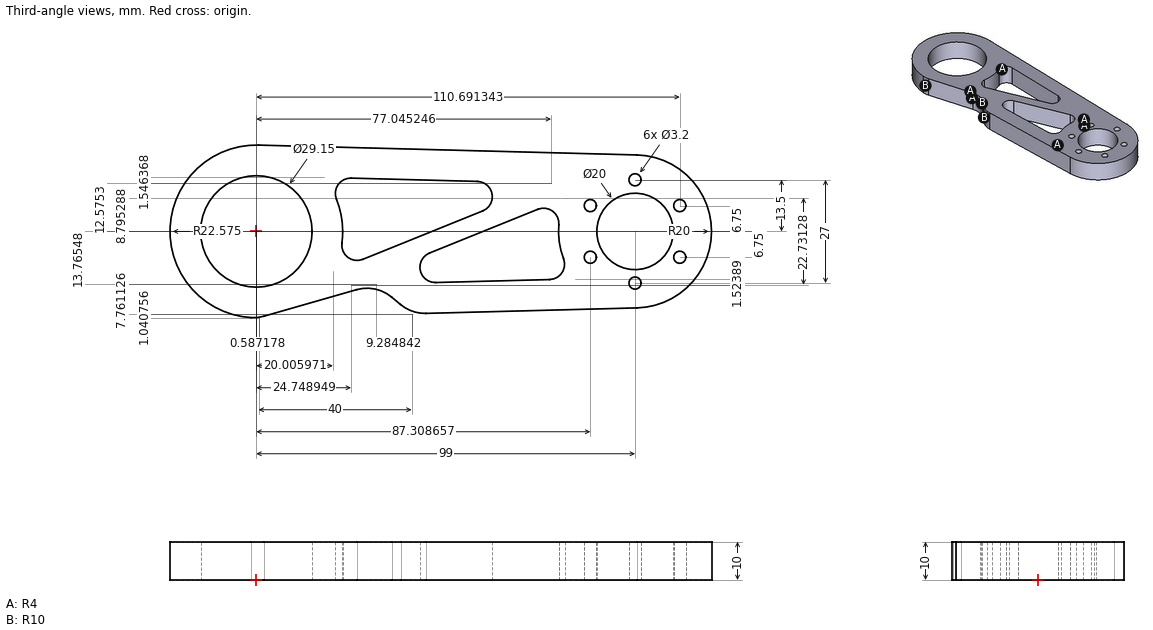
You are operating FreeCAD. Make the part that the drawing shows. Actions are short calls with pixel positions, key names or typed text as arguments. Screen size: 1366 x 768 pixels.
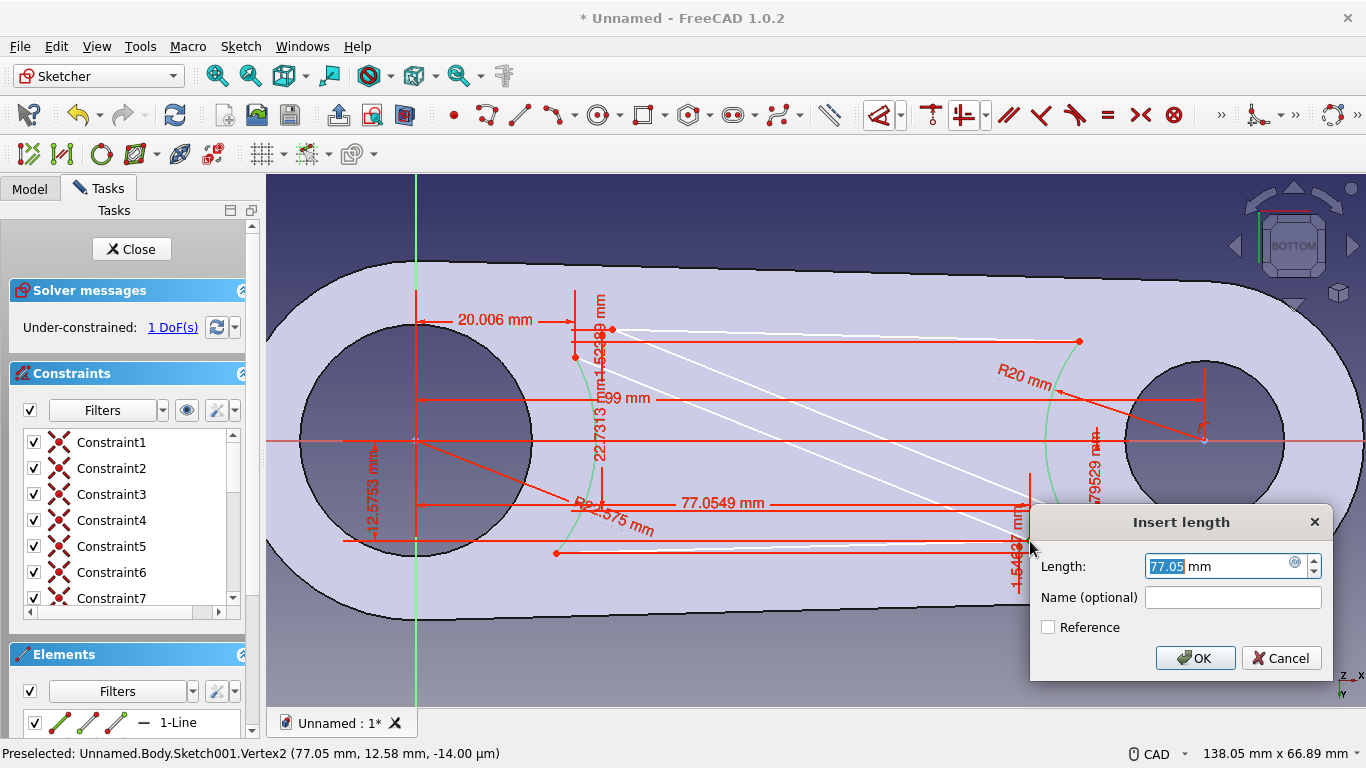
text(77.045246)
key(Return)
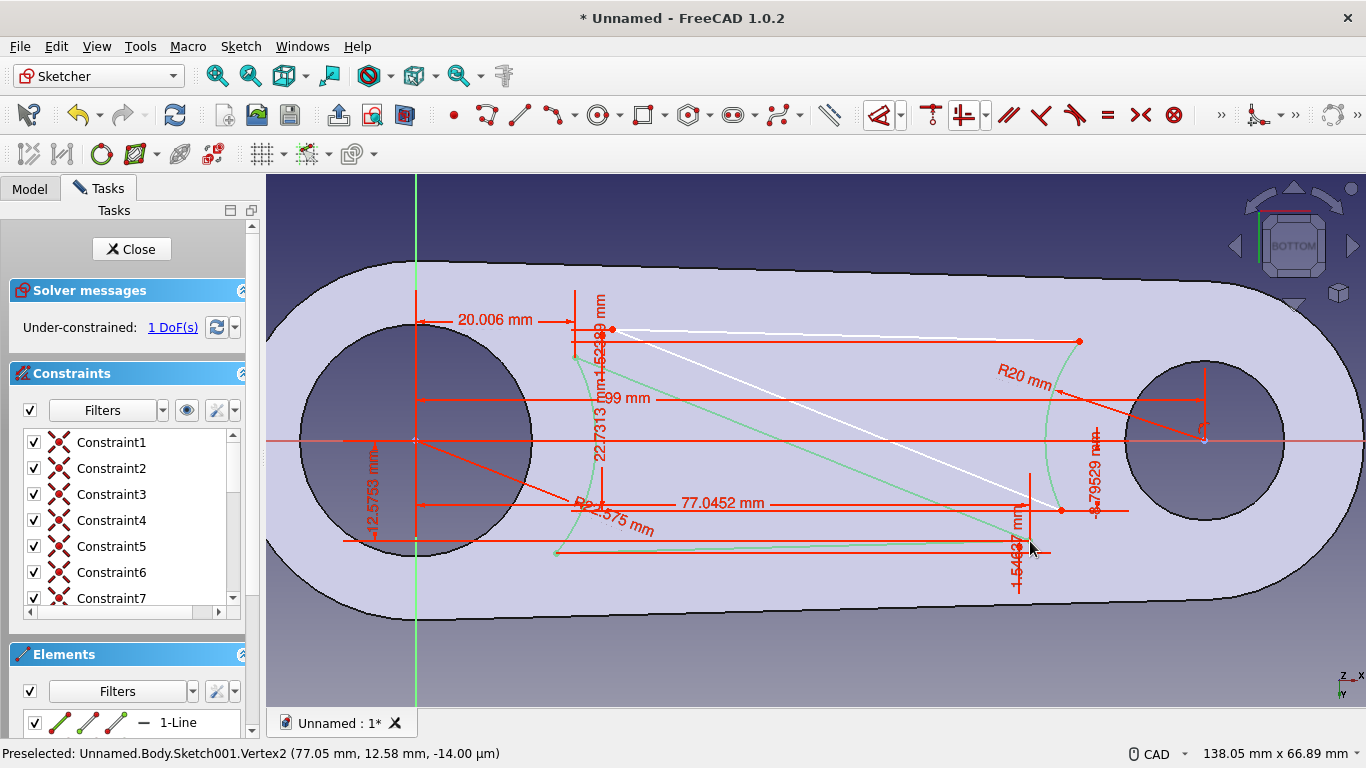
click(613, 330)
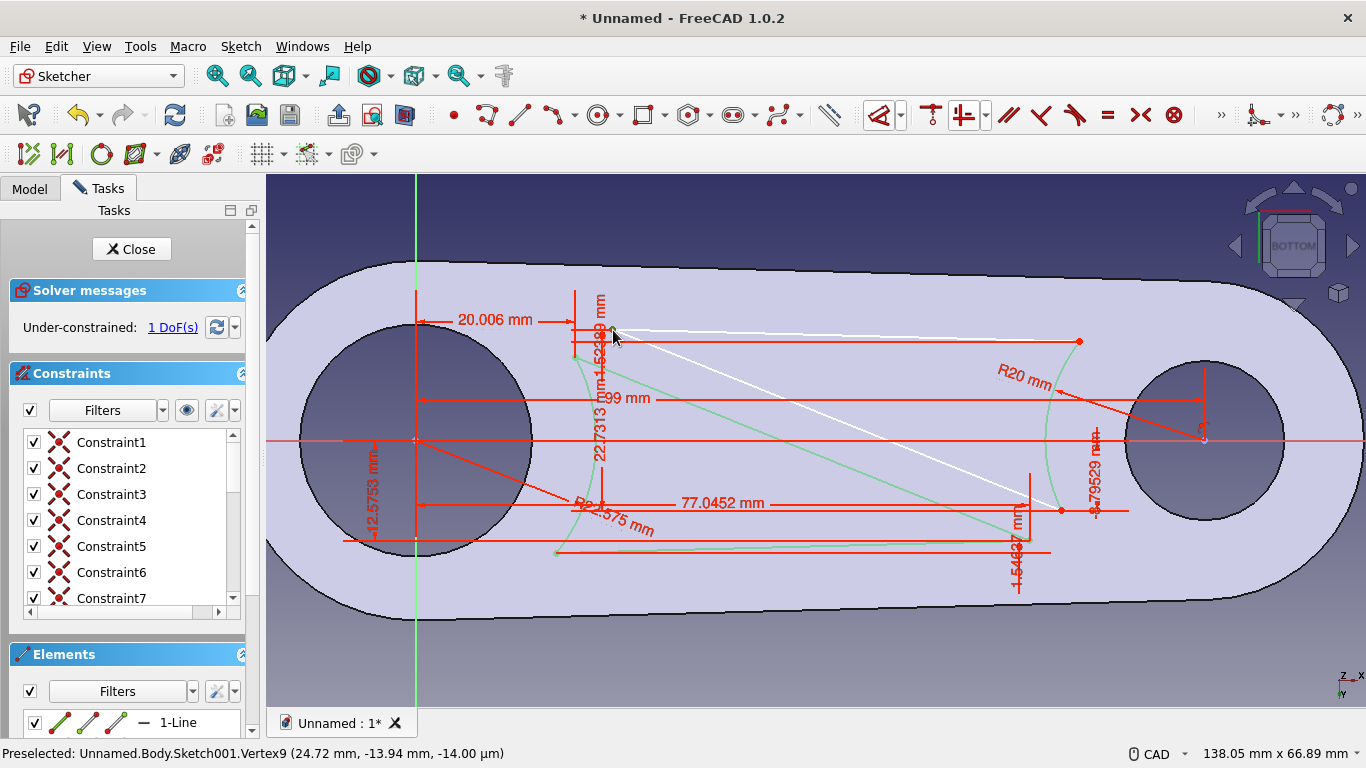
key(l)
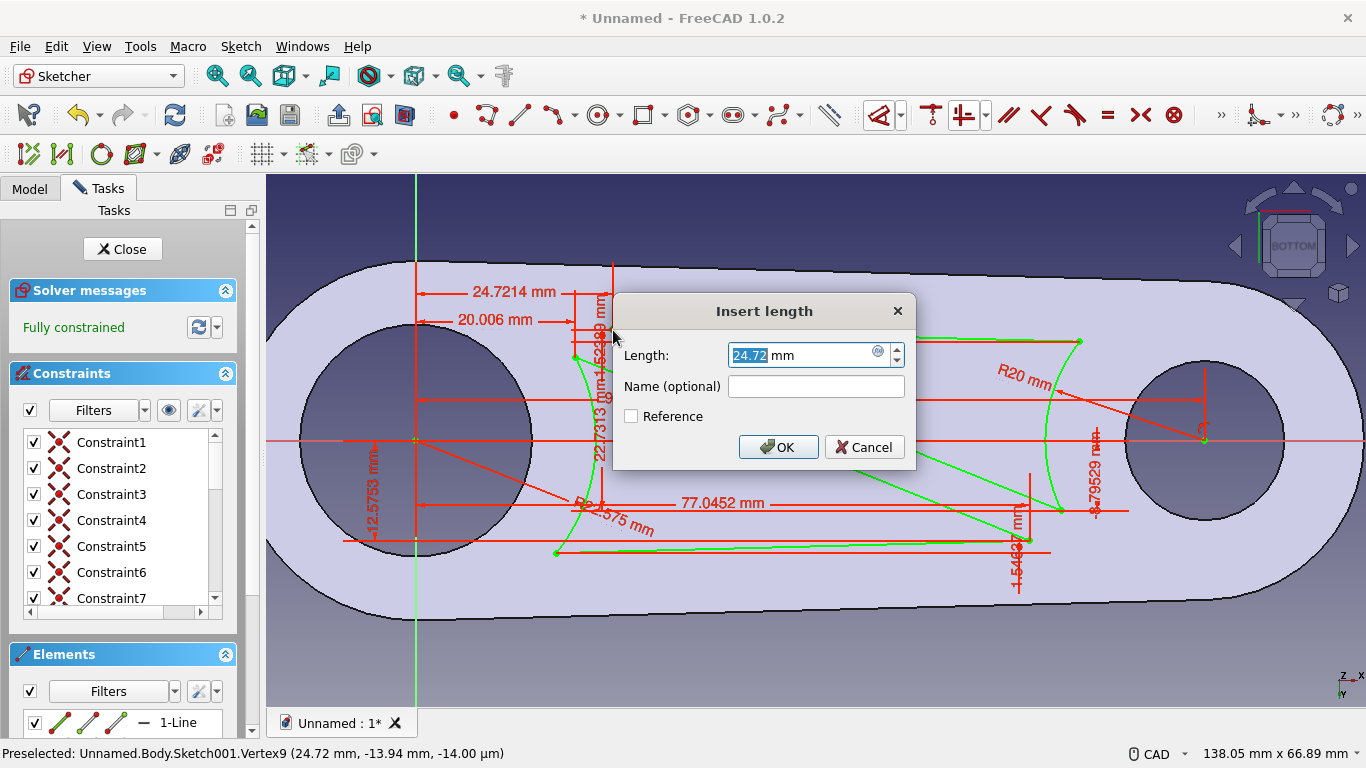
text(24.748949)
key(Return)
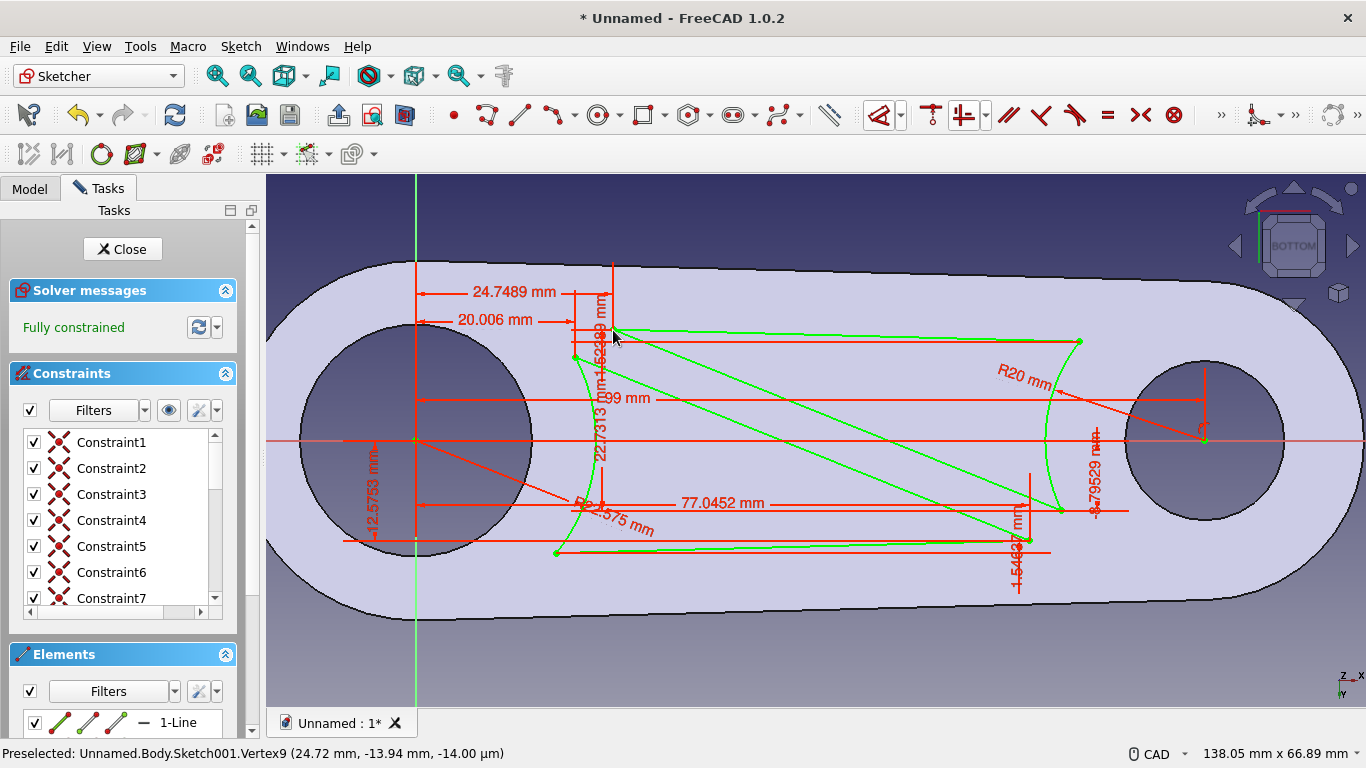
click(123, 249)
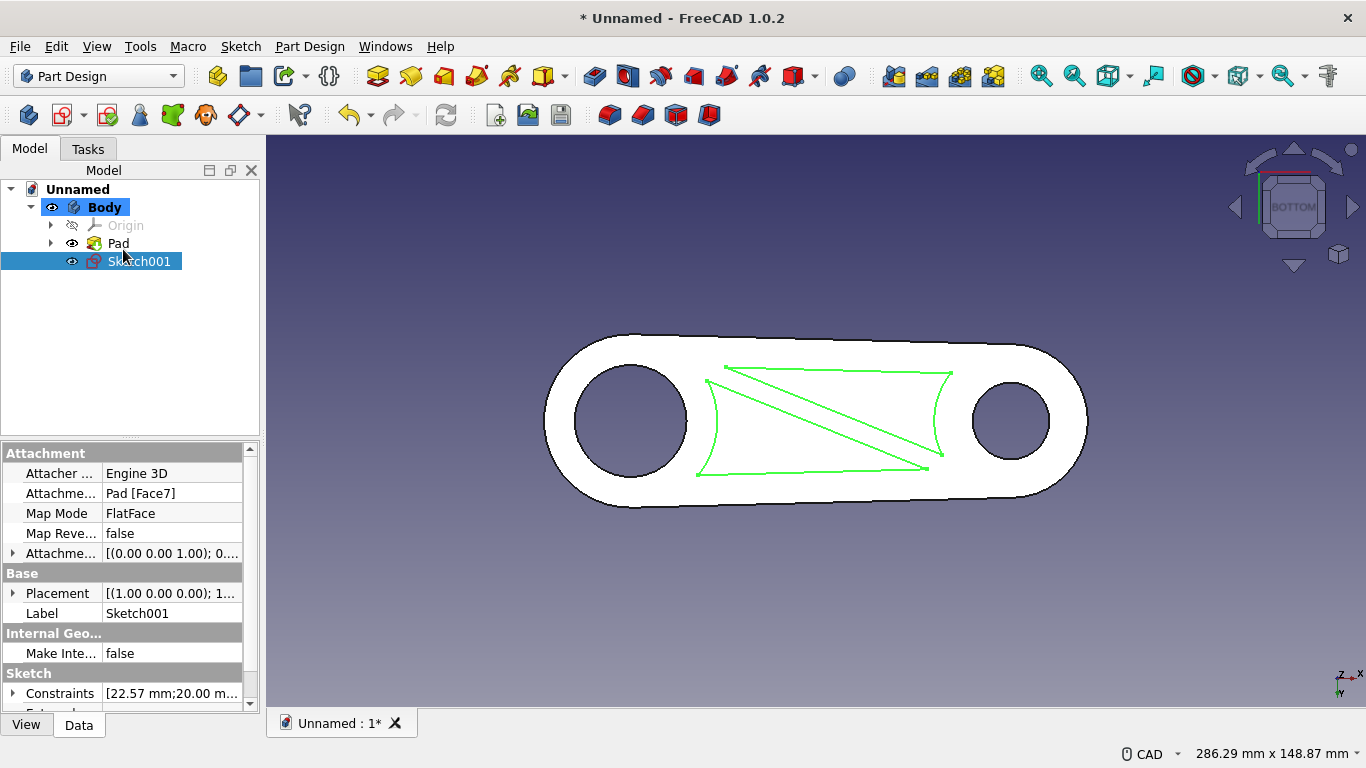
click(595, 76)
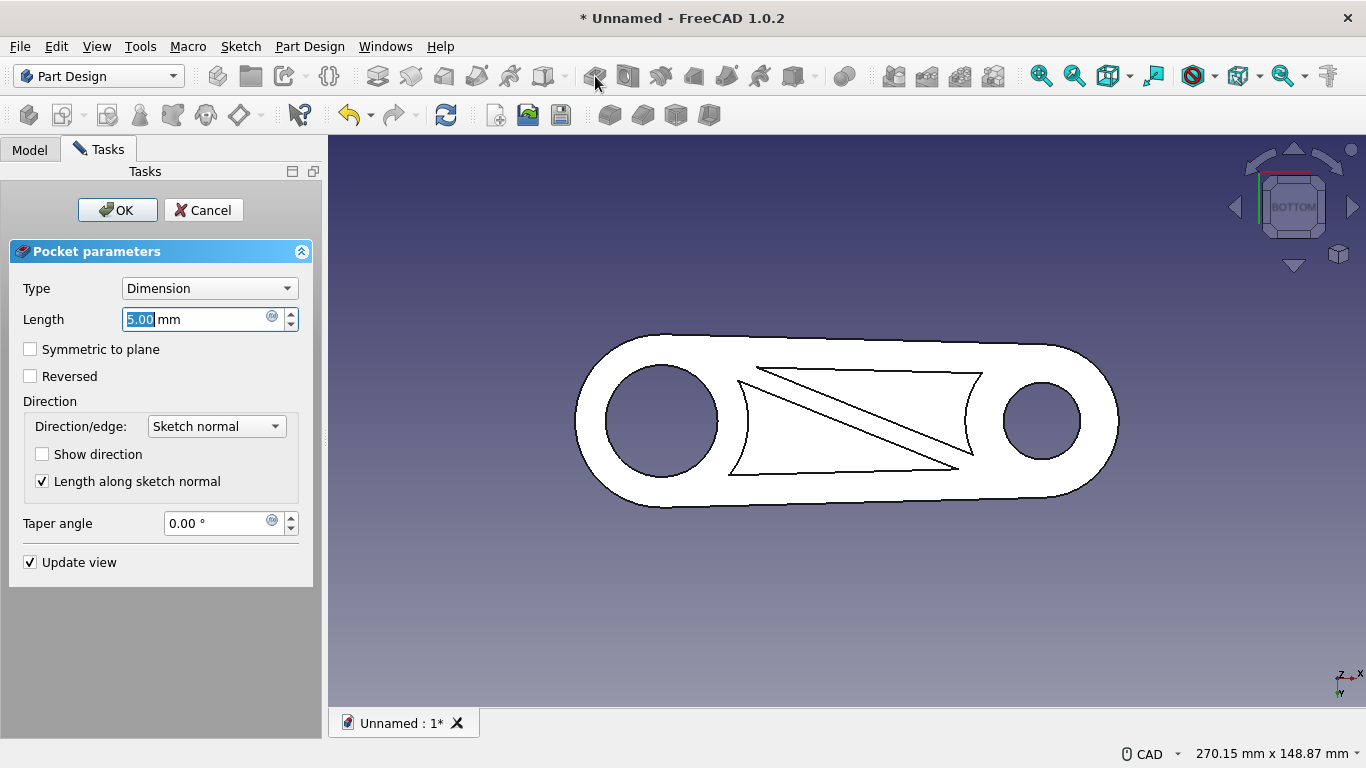
text(10)
key(Tab)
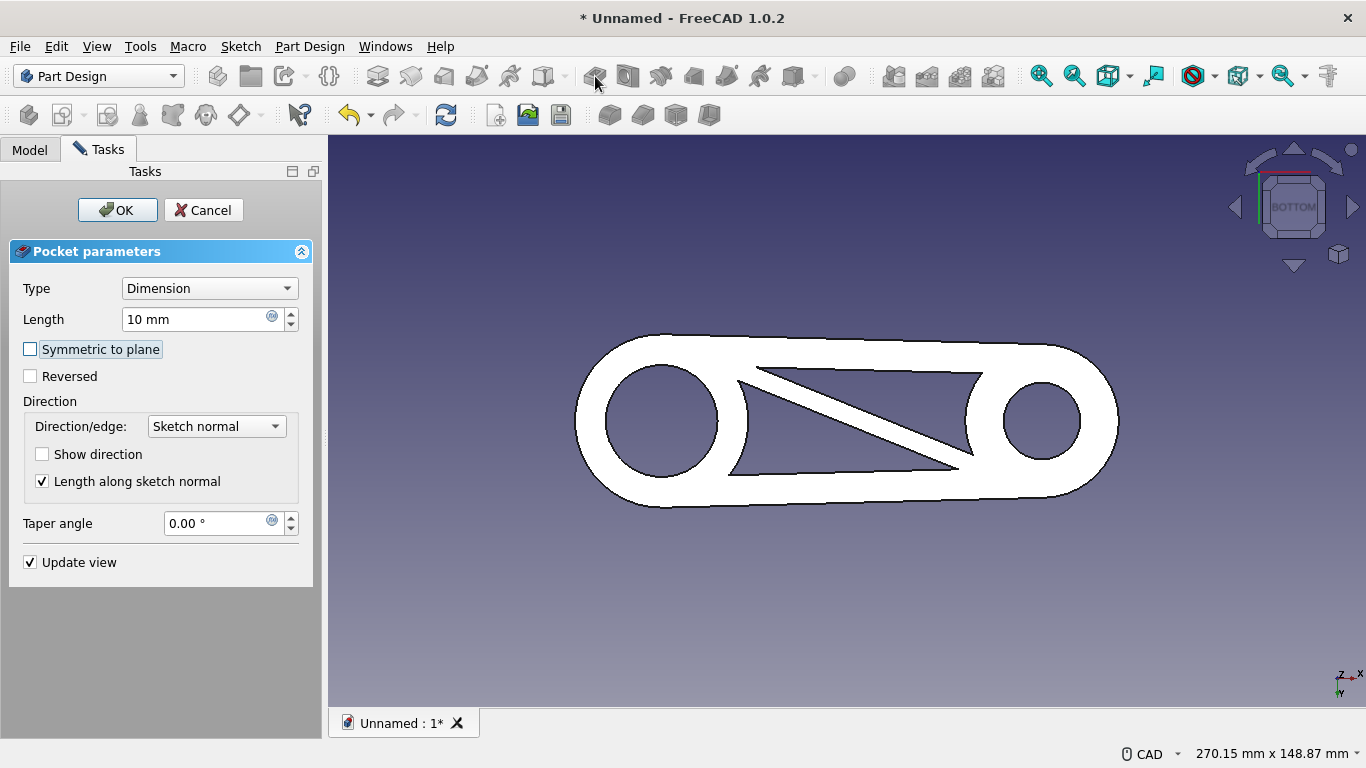
click(118, 210)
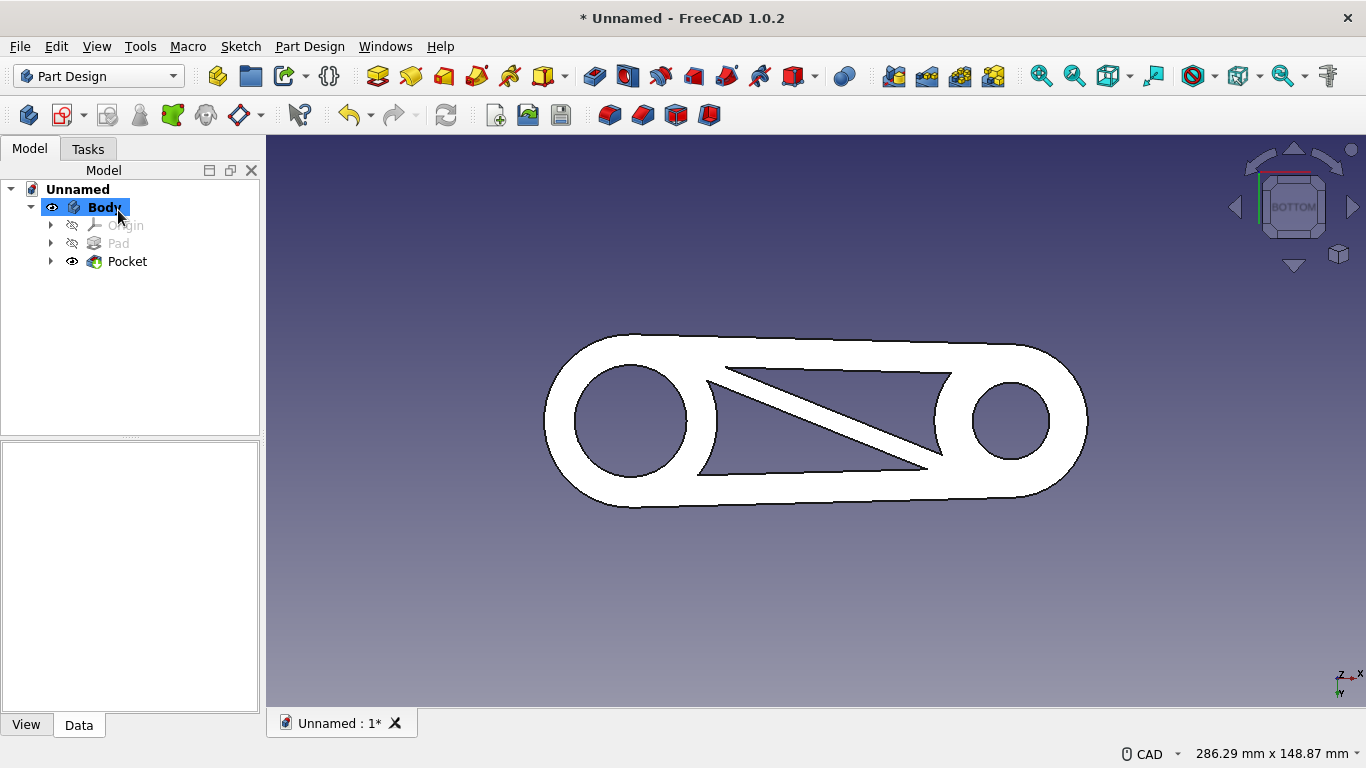
key(0)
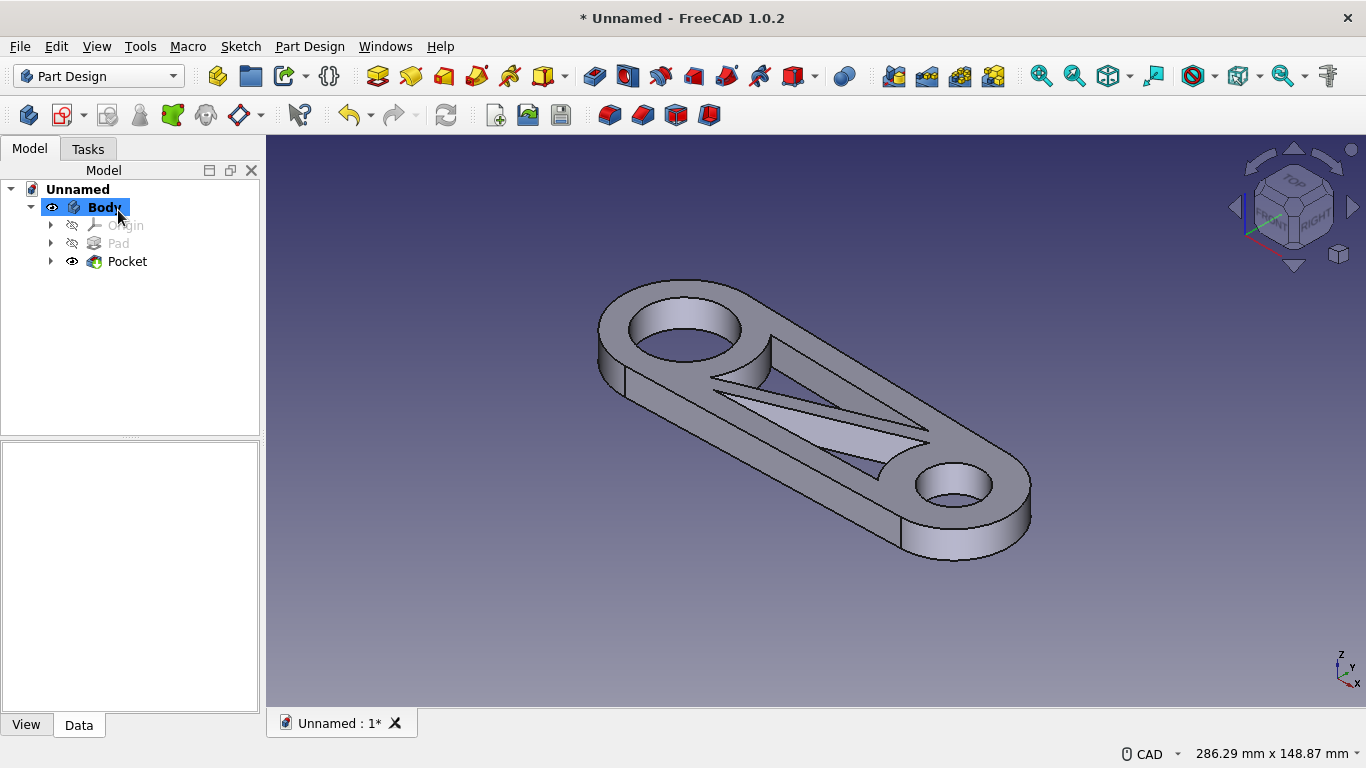
key(2)